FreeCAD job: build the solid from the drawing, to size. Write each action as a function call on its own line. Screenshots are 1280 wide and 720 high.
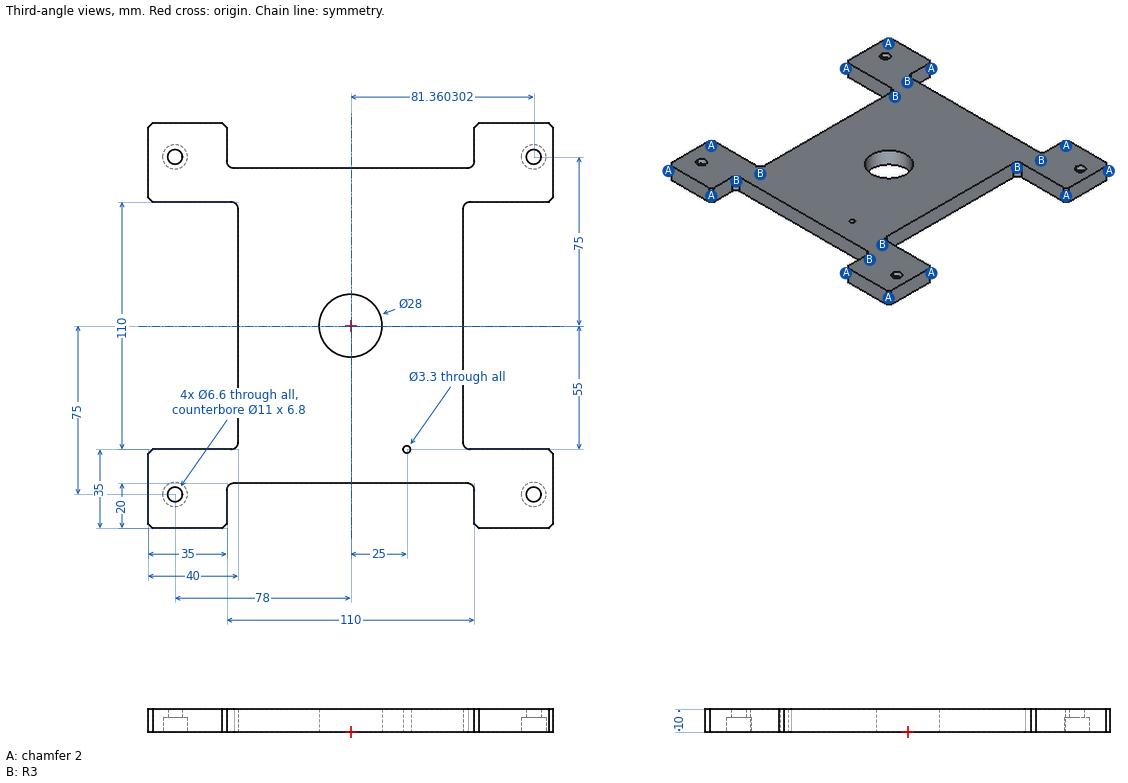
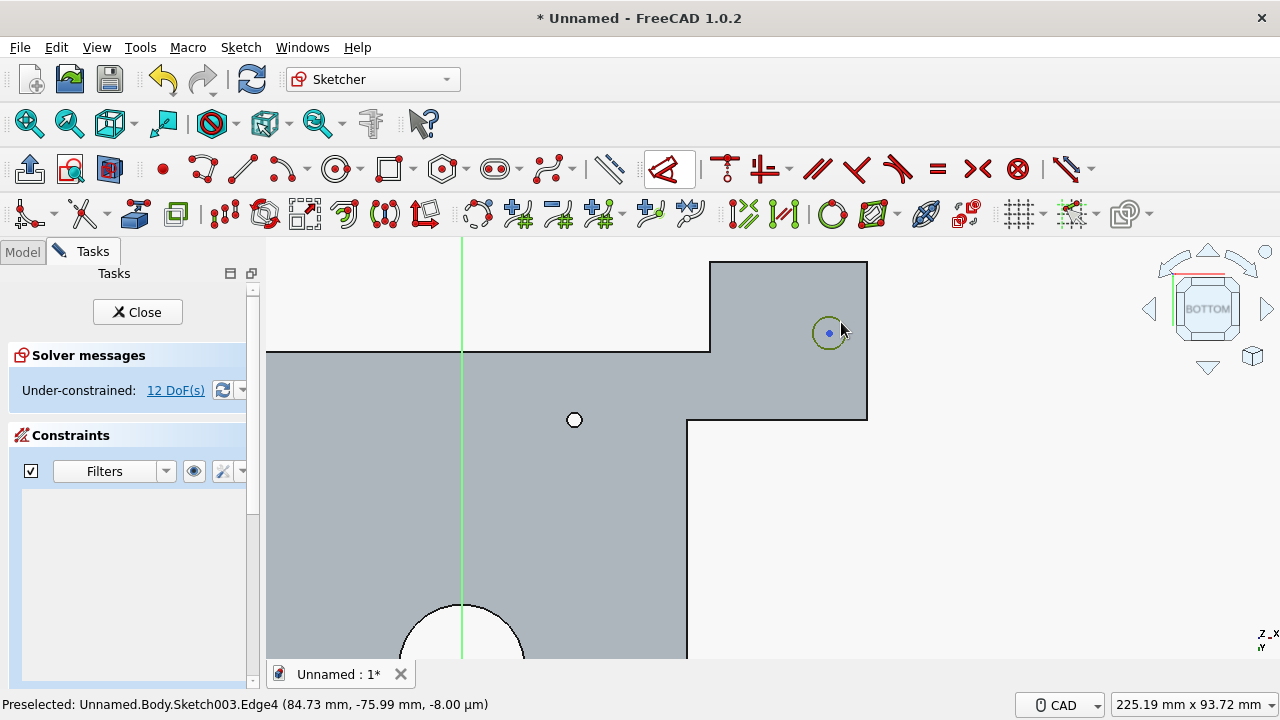
click(938, 170)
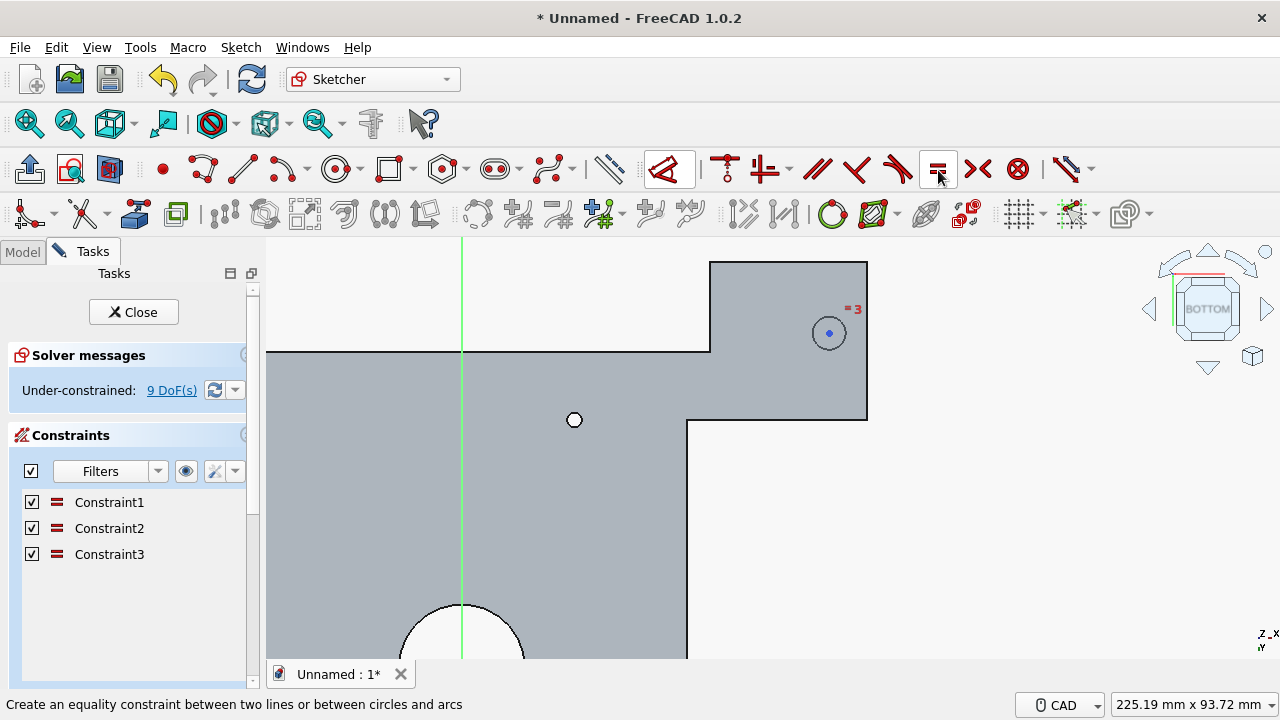
scroll(841, 320, down, 5)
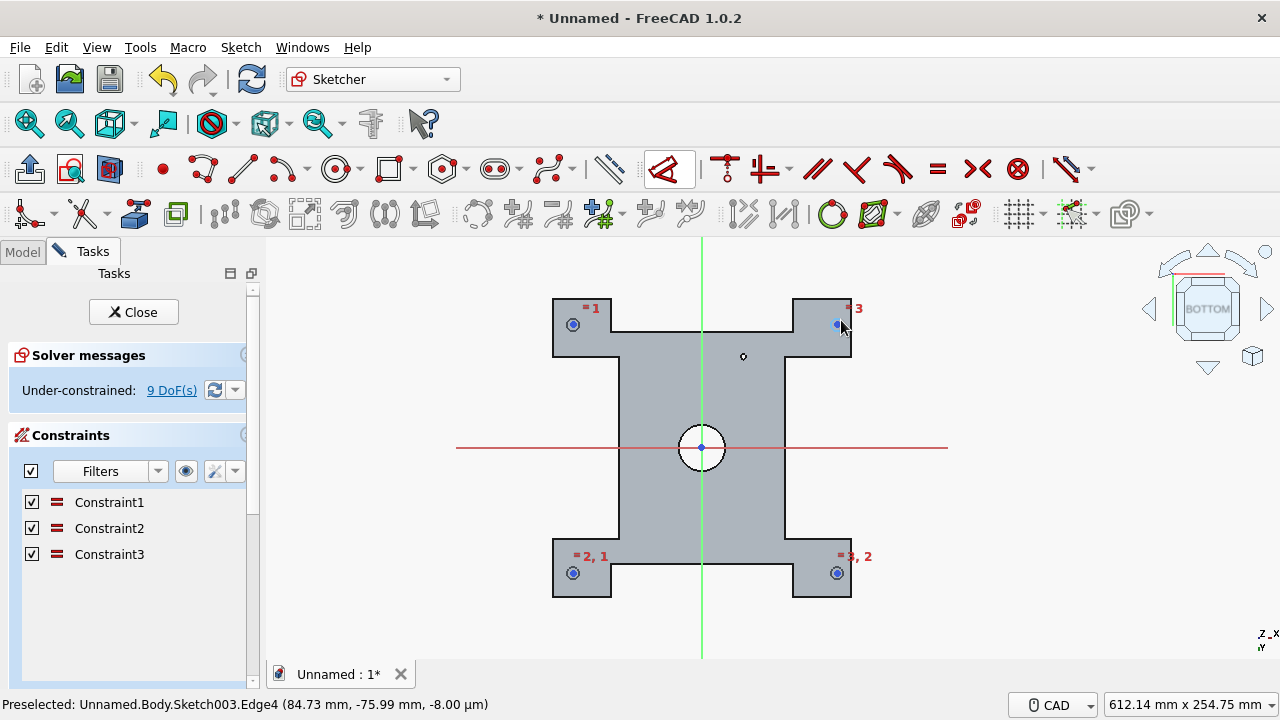
click(573, 325)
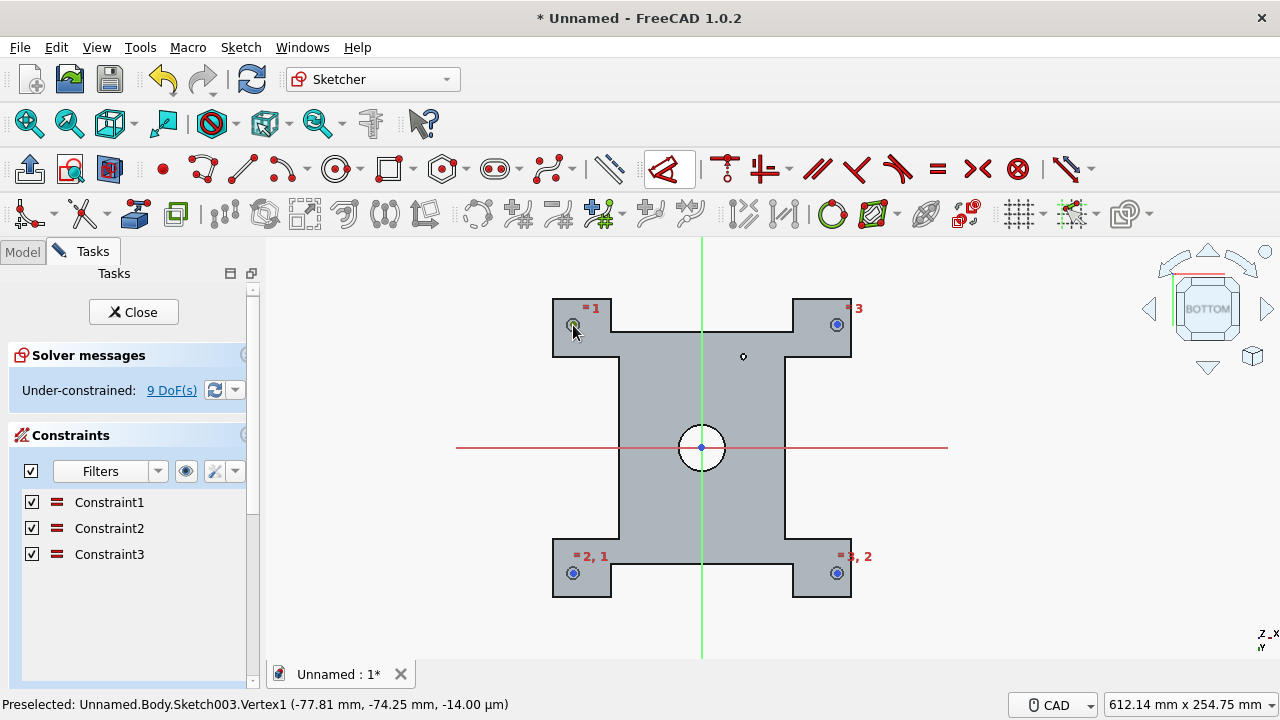
click(573, 573)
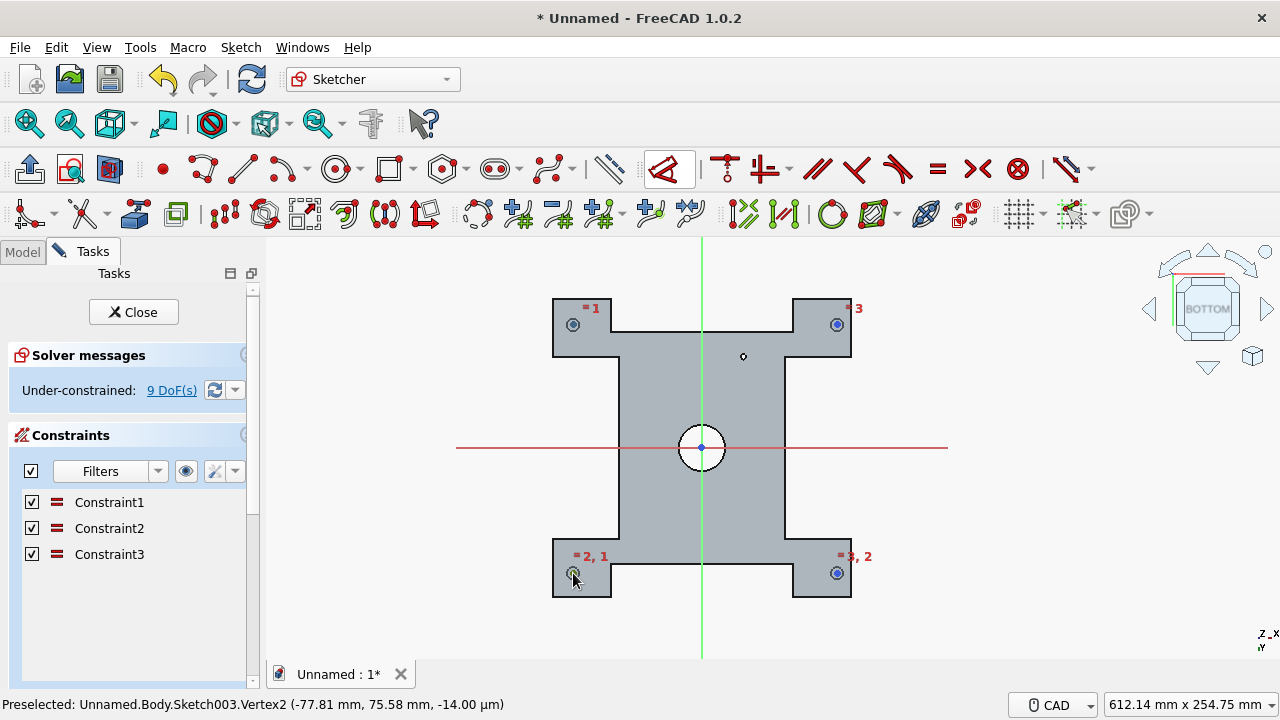
click(470, 448)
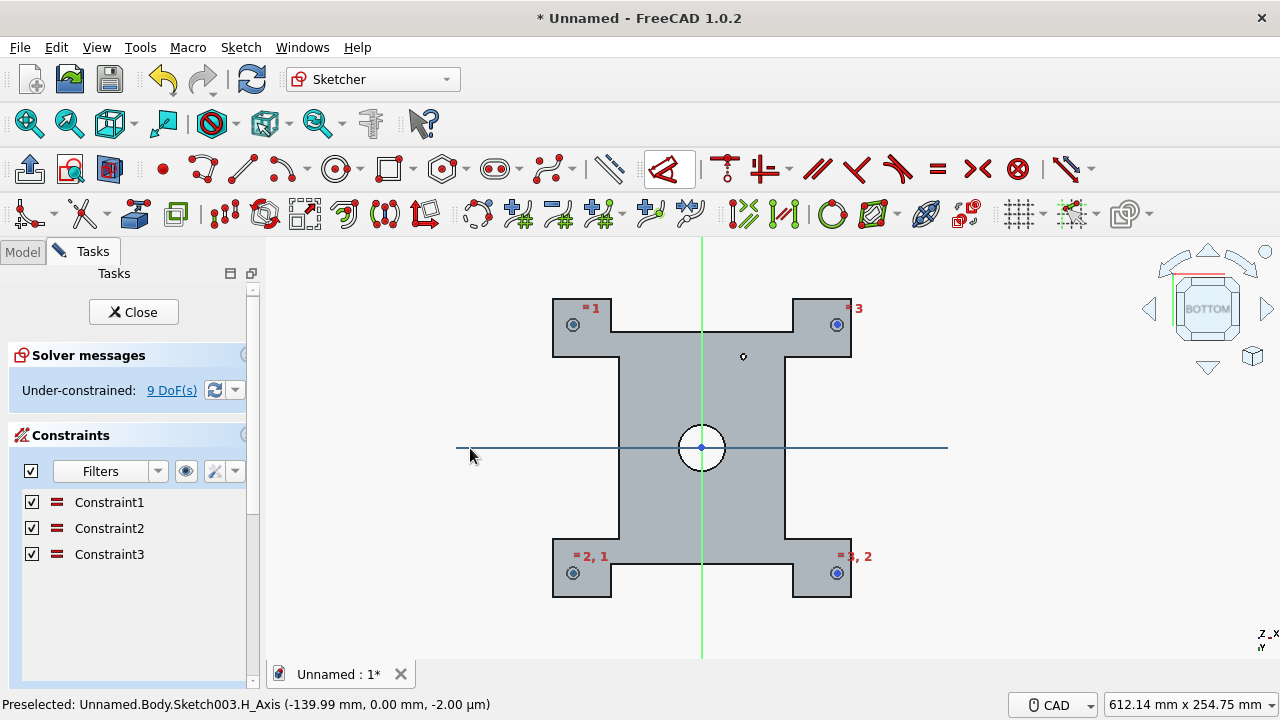
click(978, 170)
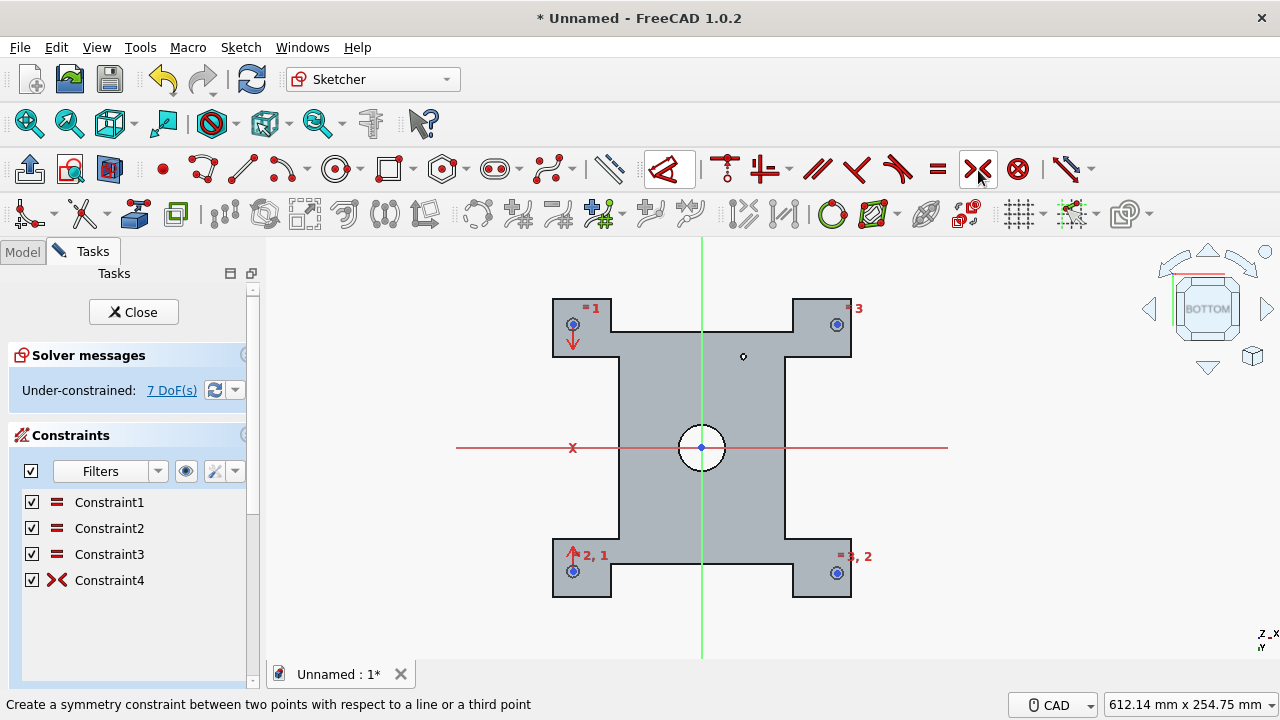
click(837, 573)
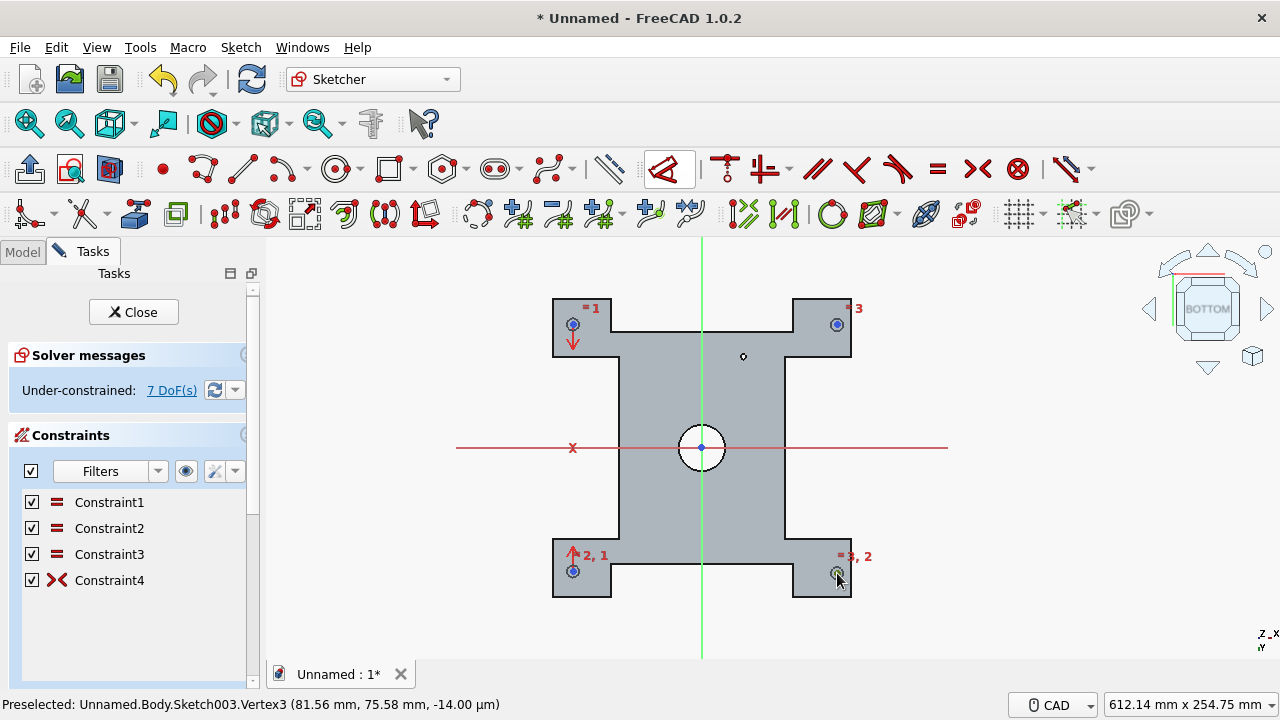
click(837, 325)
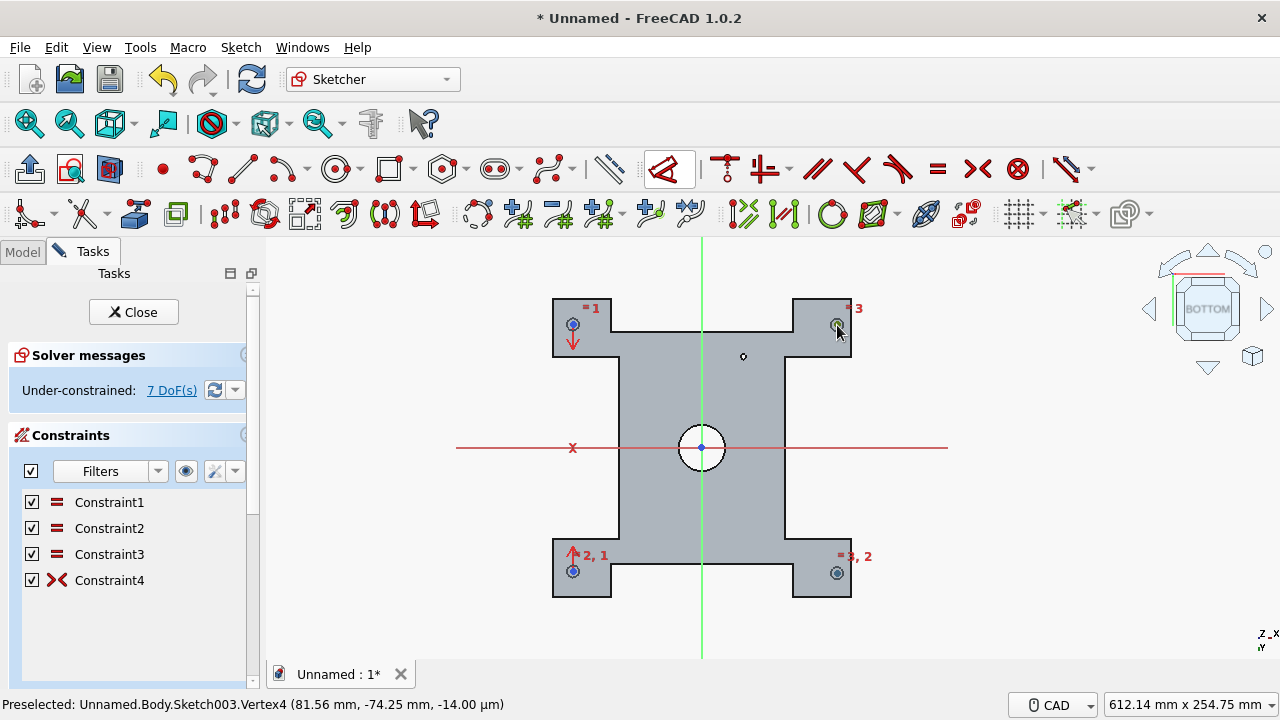
click(470, 448)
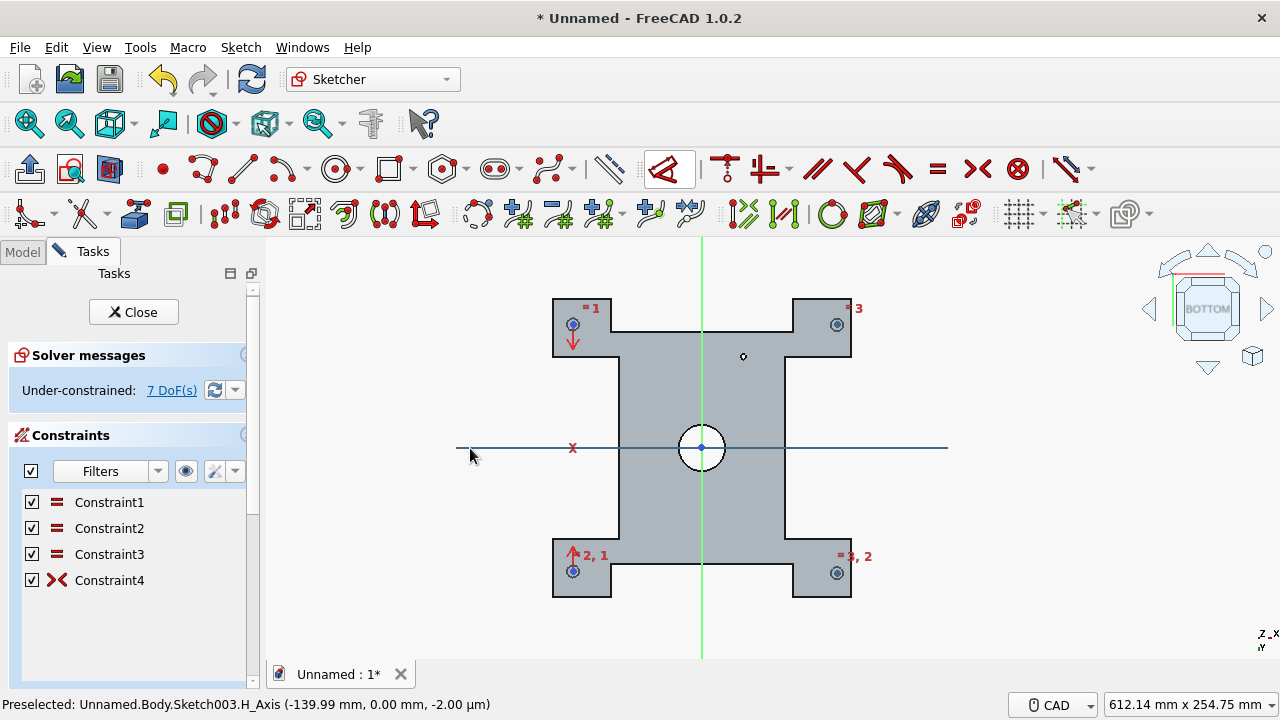
click(978, 170)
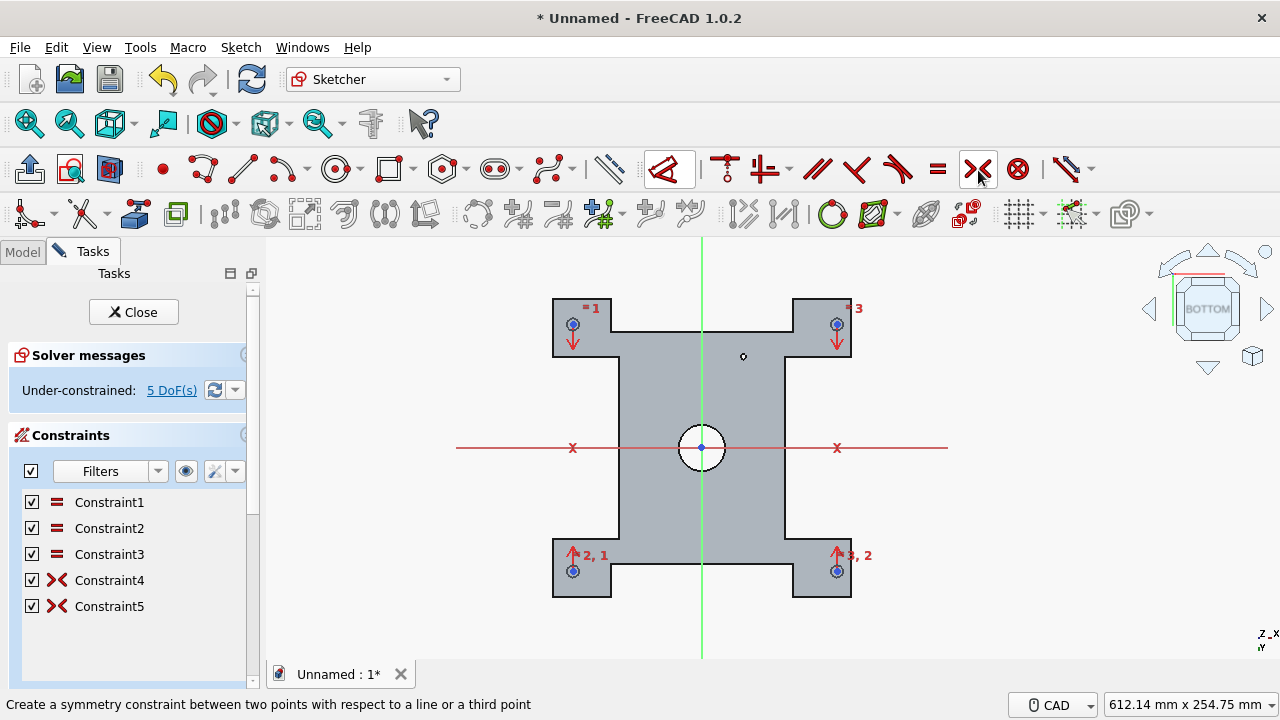
scroll(577, 320, up, 7)